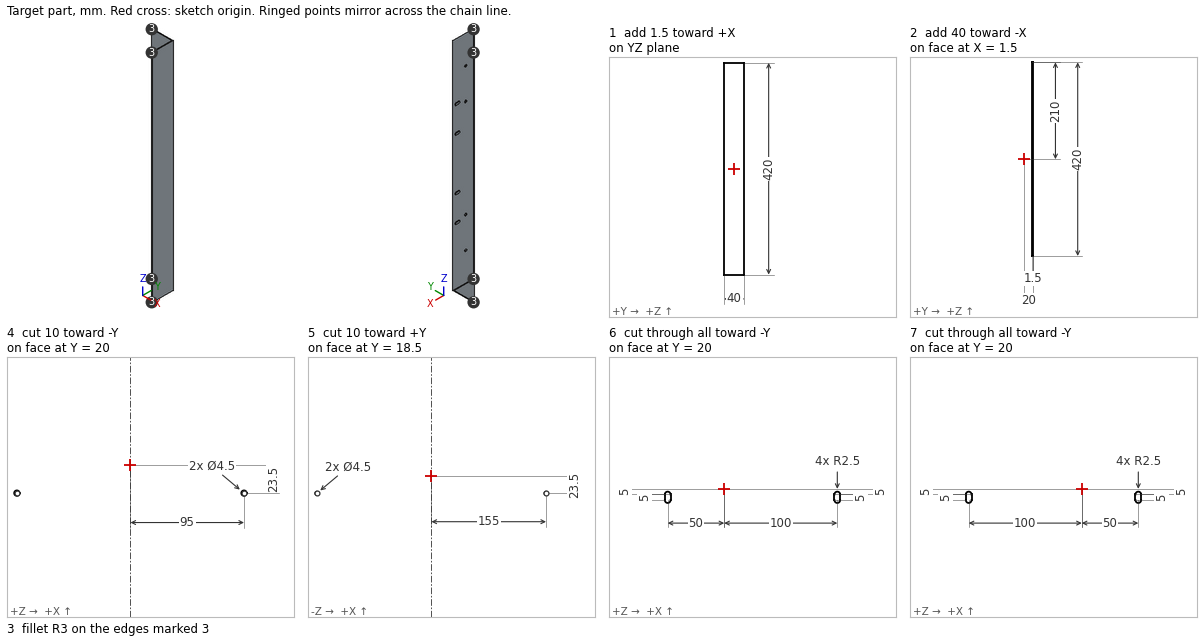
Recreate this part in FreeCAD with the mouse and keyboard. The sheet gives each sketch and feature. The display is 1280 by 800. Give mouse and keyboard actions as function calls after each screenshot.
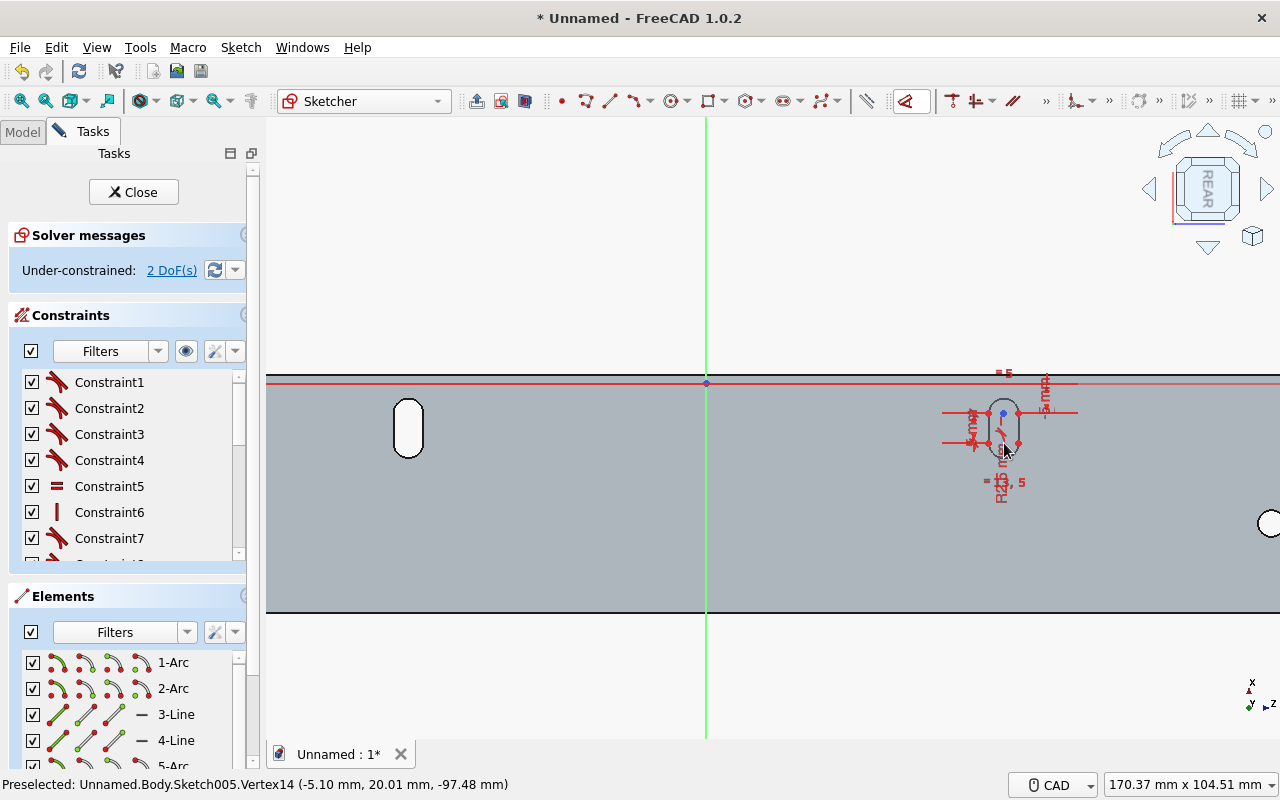
click(1004, 443)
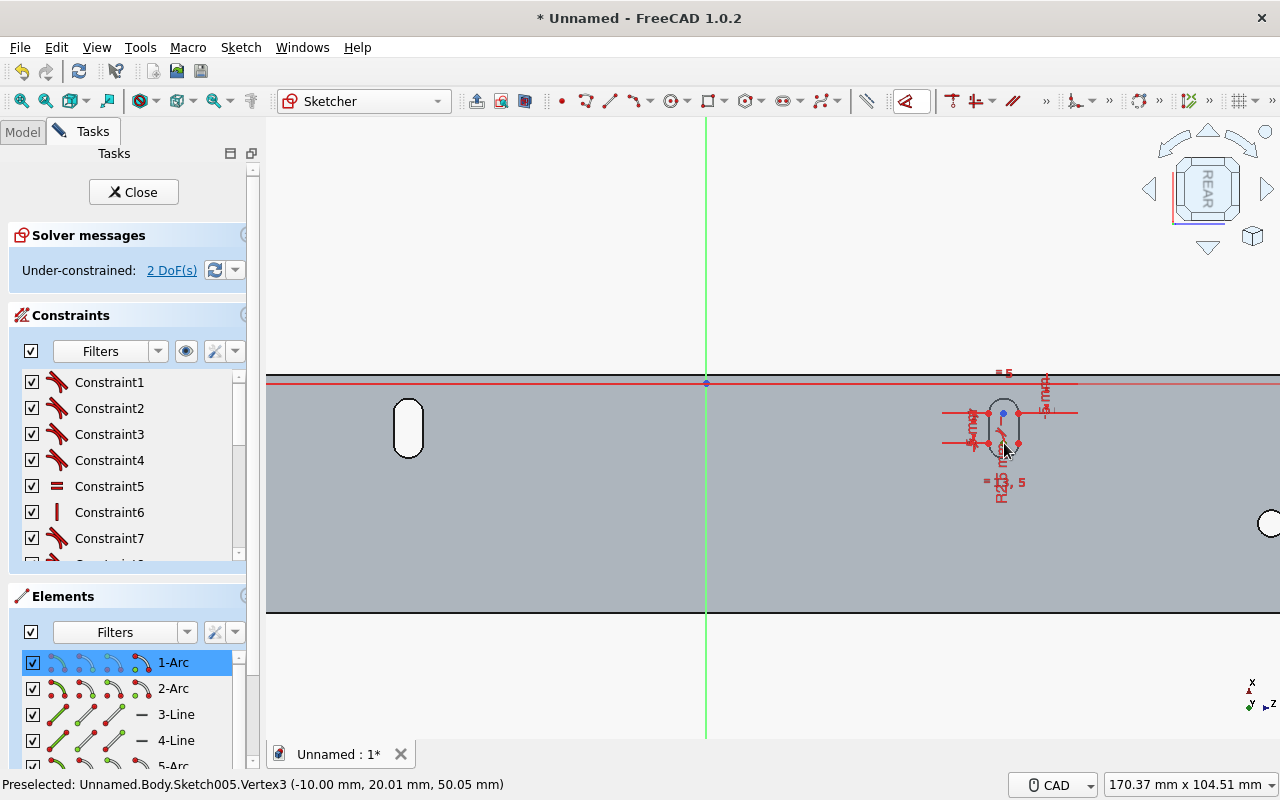
click(924, 102)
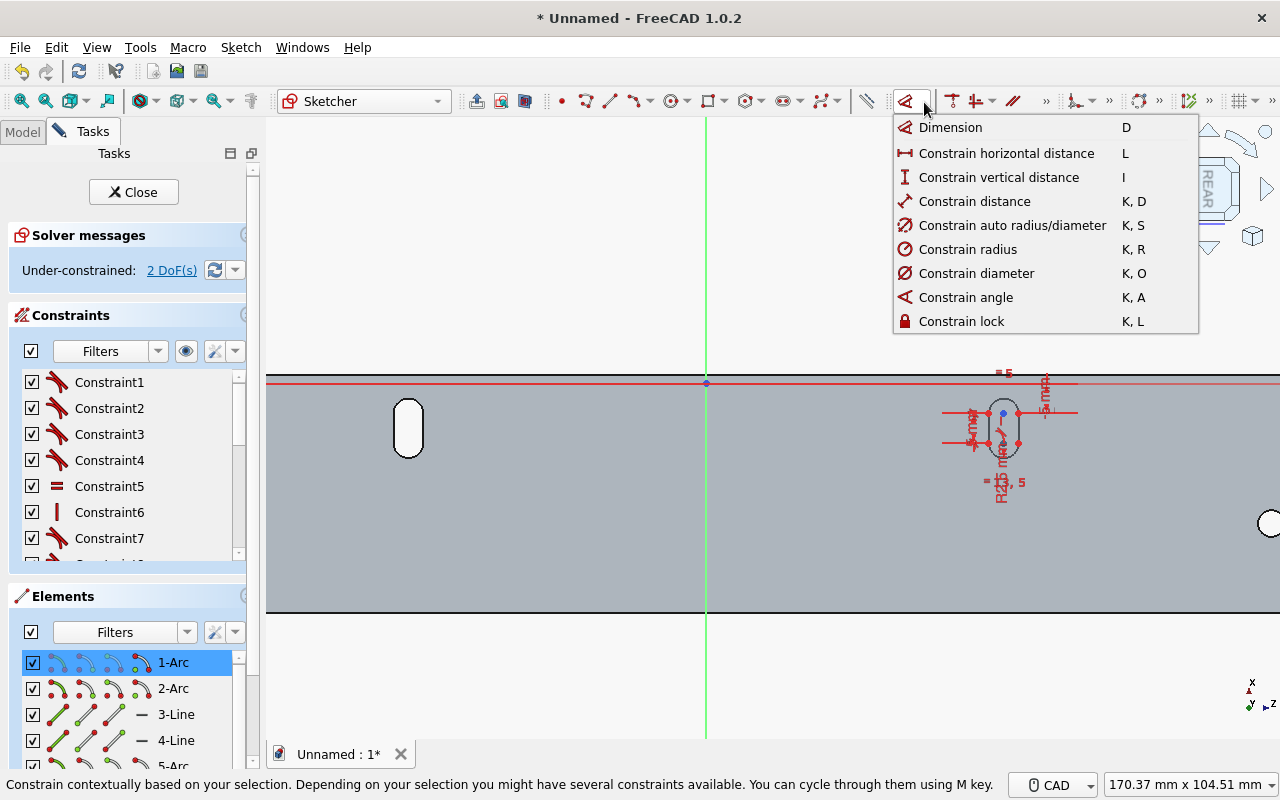
click(1046, 153)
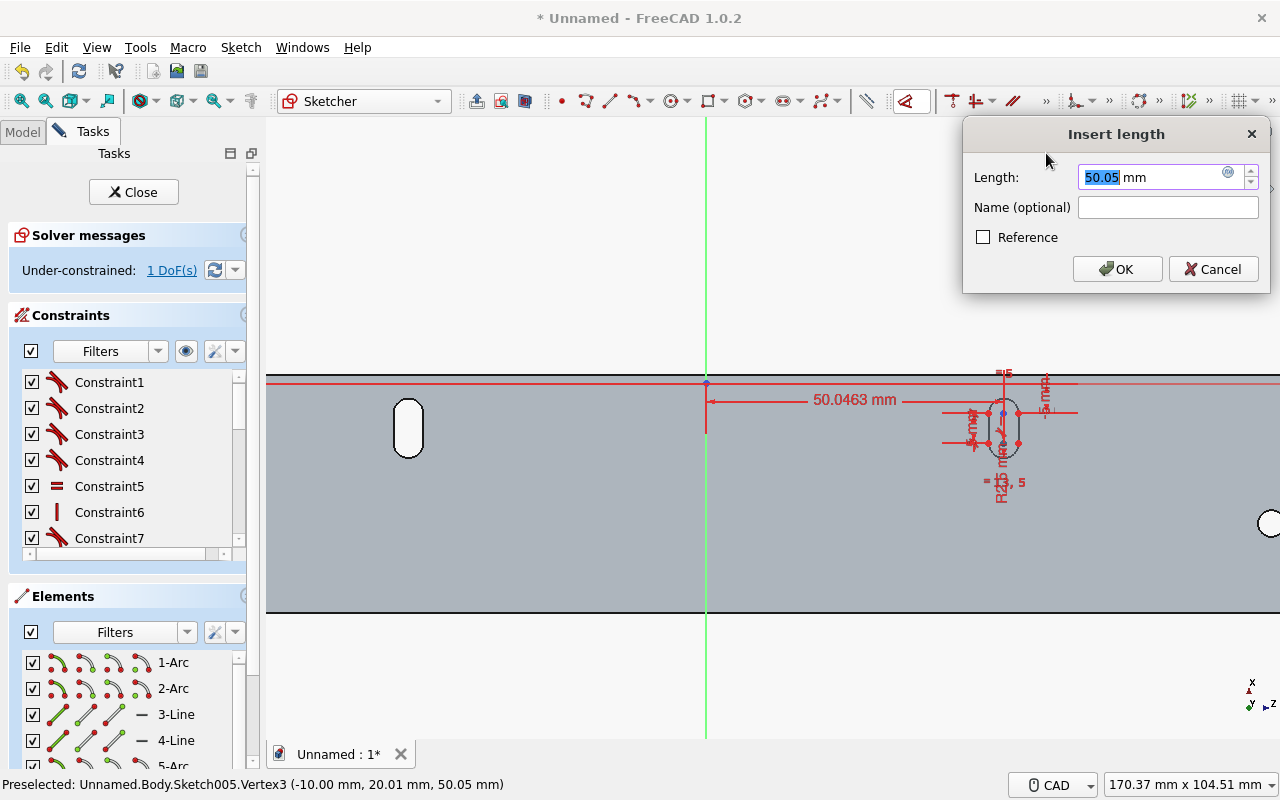
text(50)
key(Return)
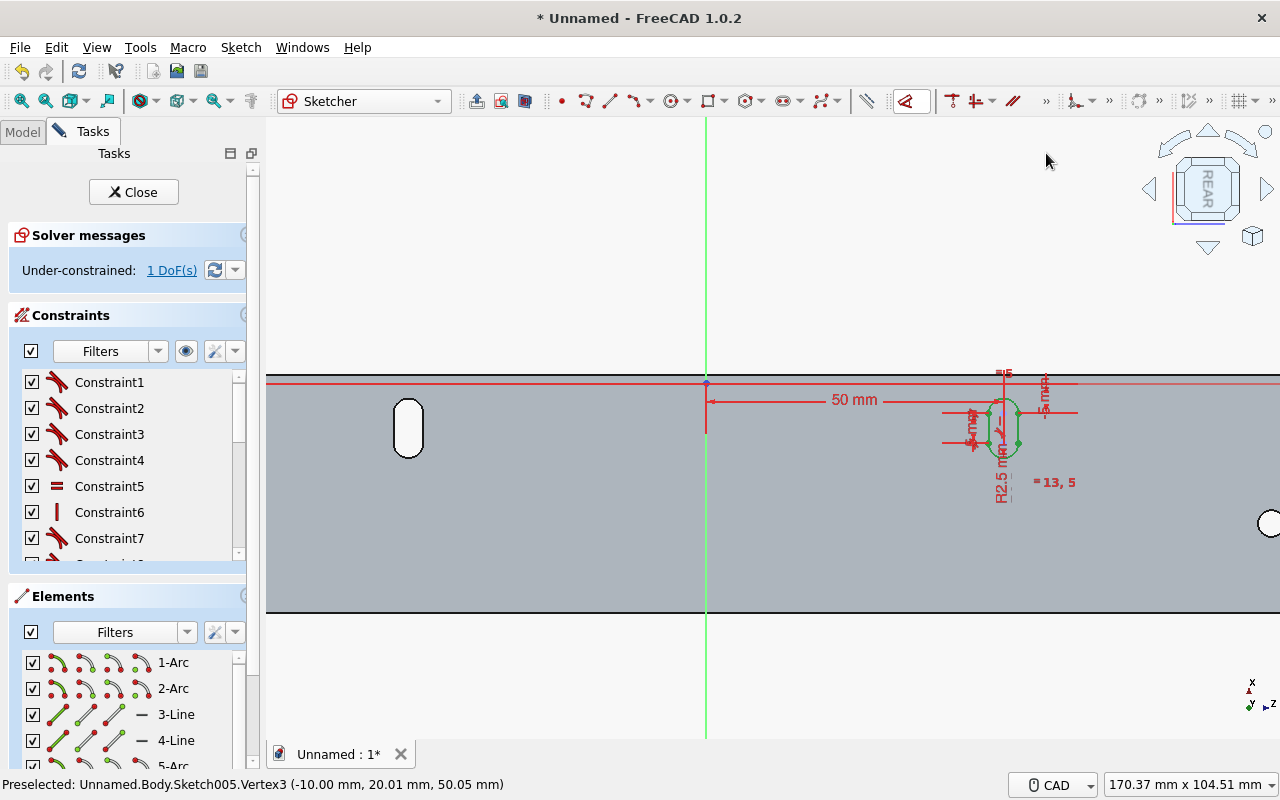
scroll(1004, 442, down, 2)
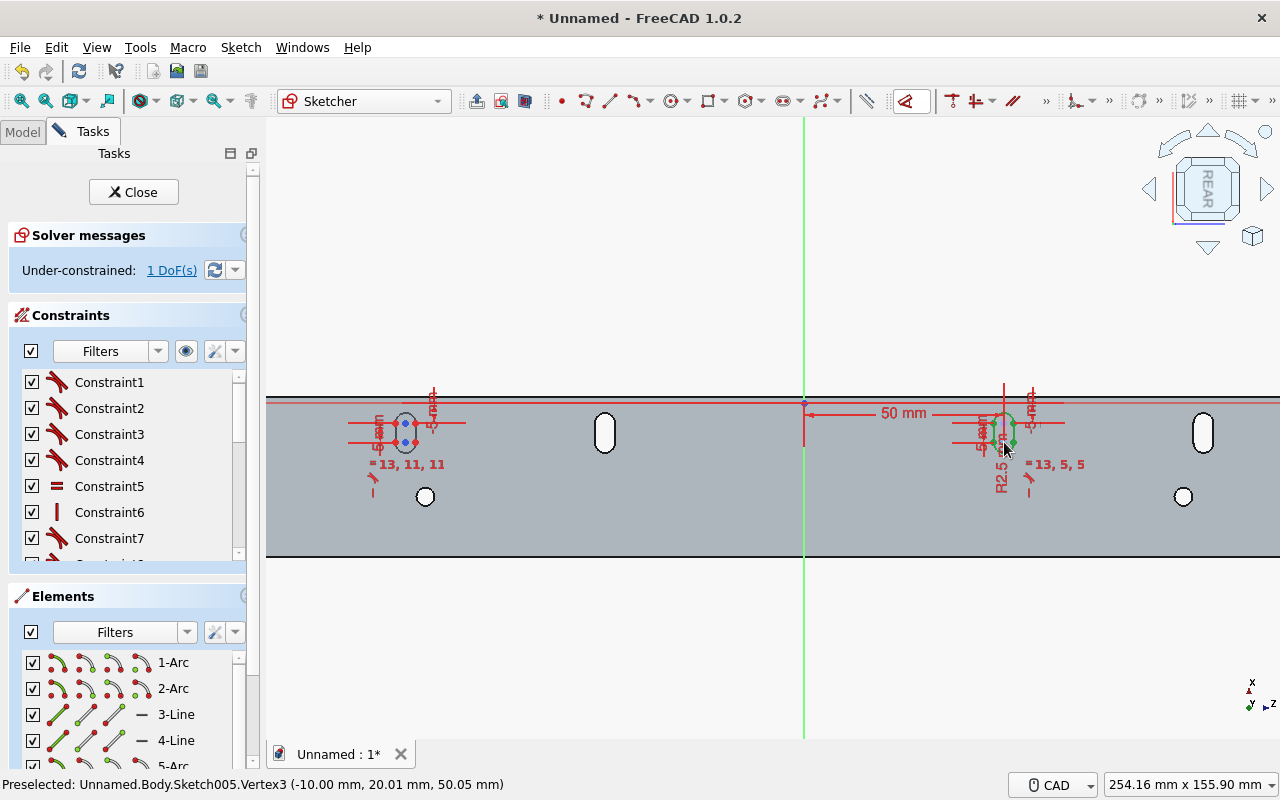
scroll(406, 443, up, 2)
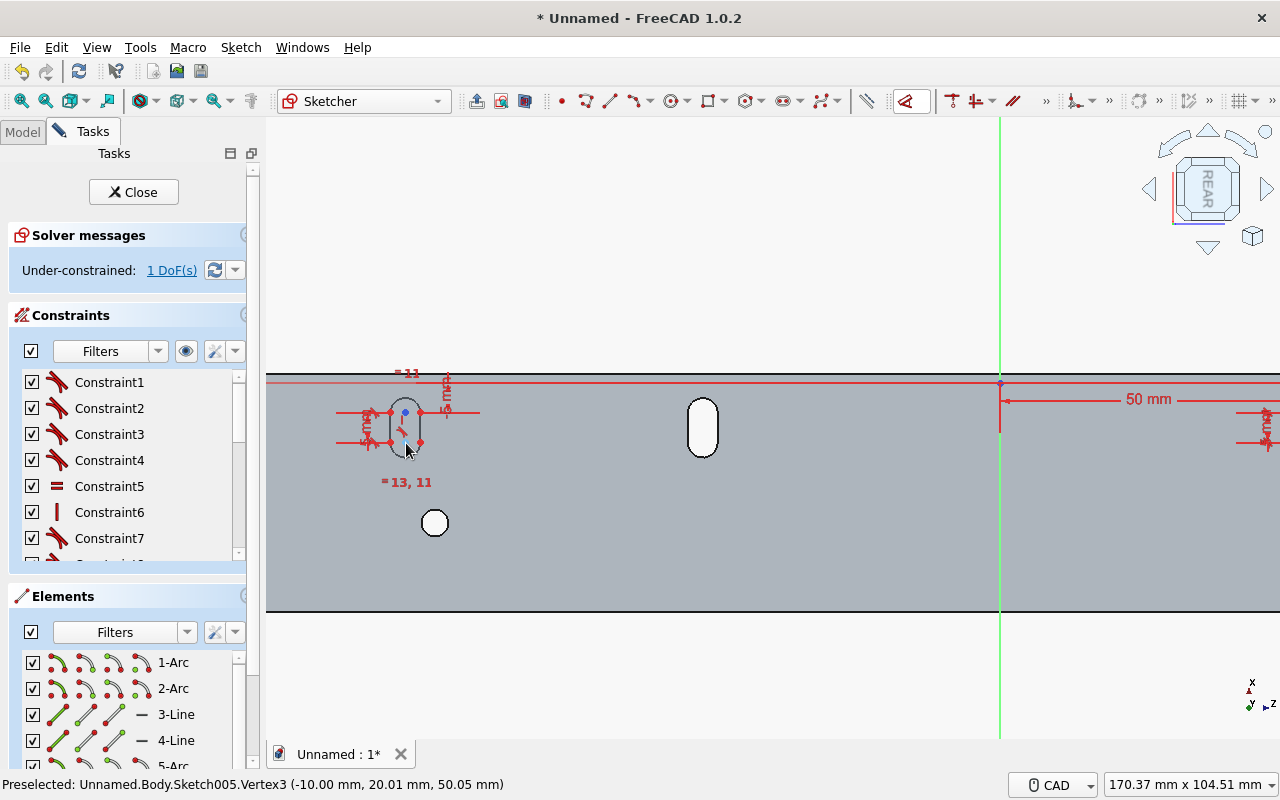
click(405, 443)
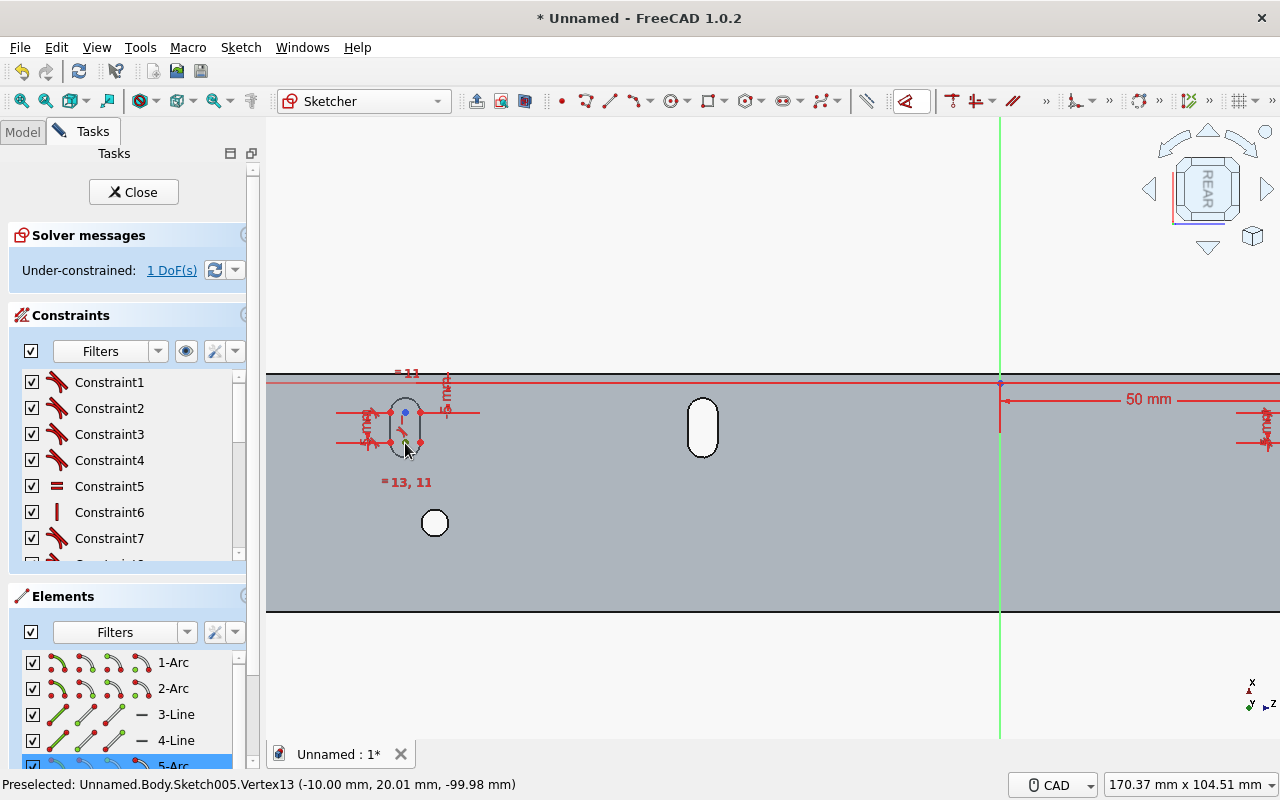
key(l)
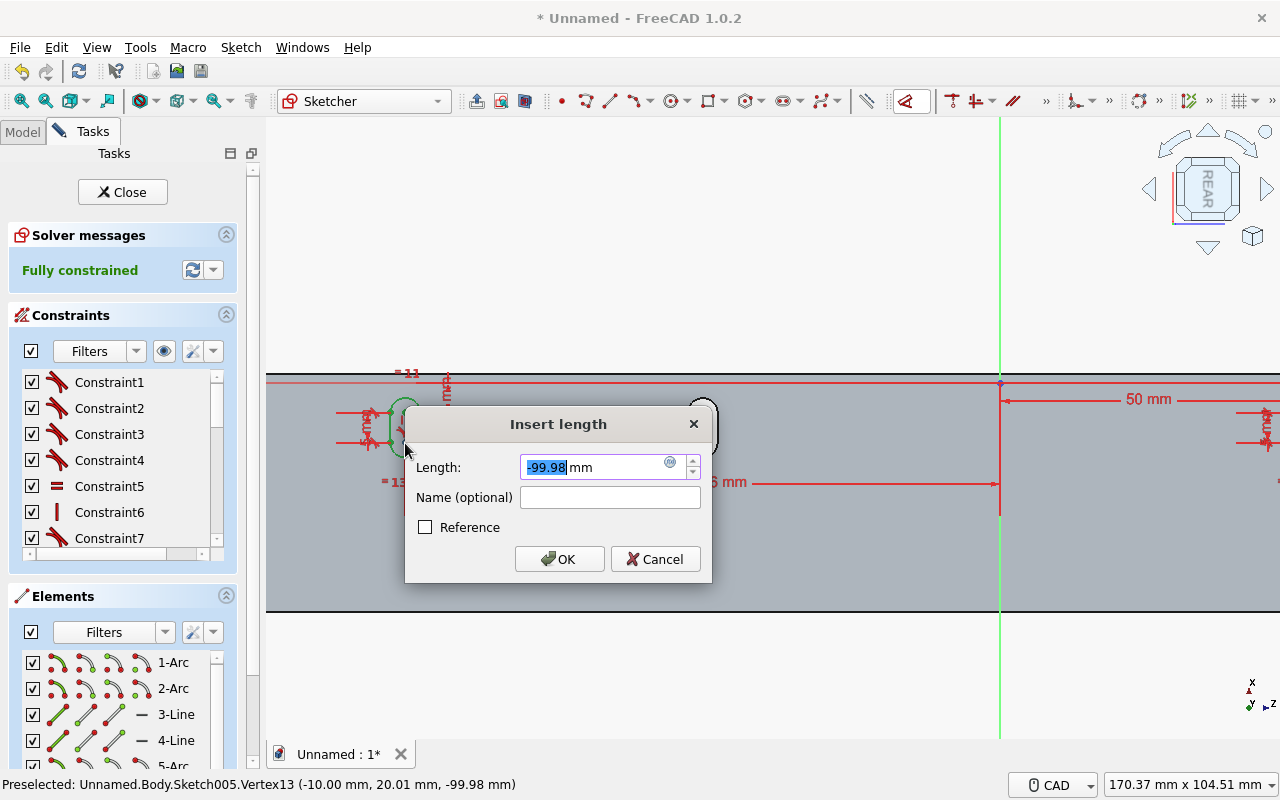
text(-100)
key(Return)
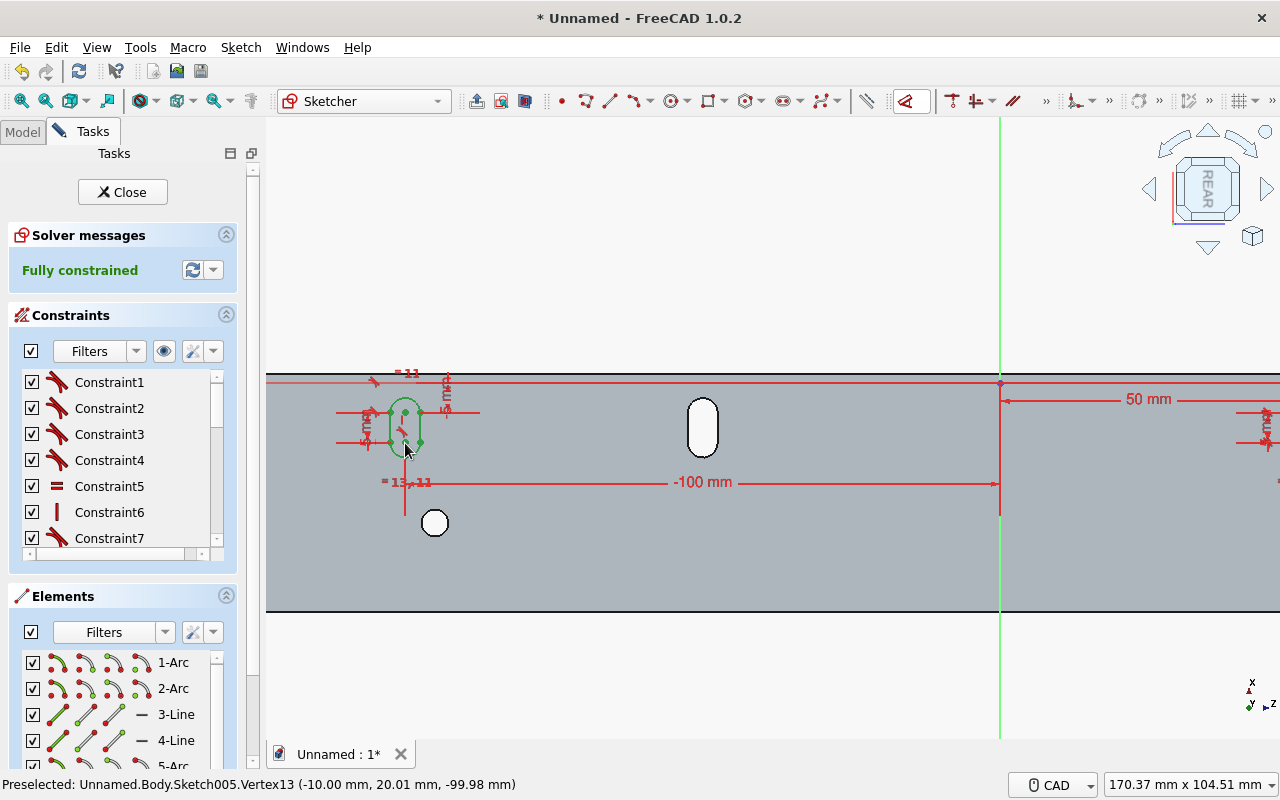
click(123, 192)